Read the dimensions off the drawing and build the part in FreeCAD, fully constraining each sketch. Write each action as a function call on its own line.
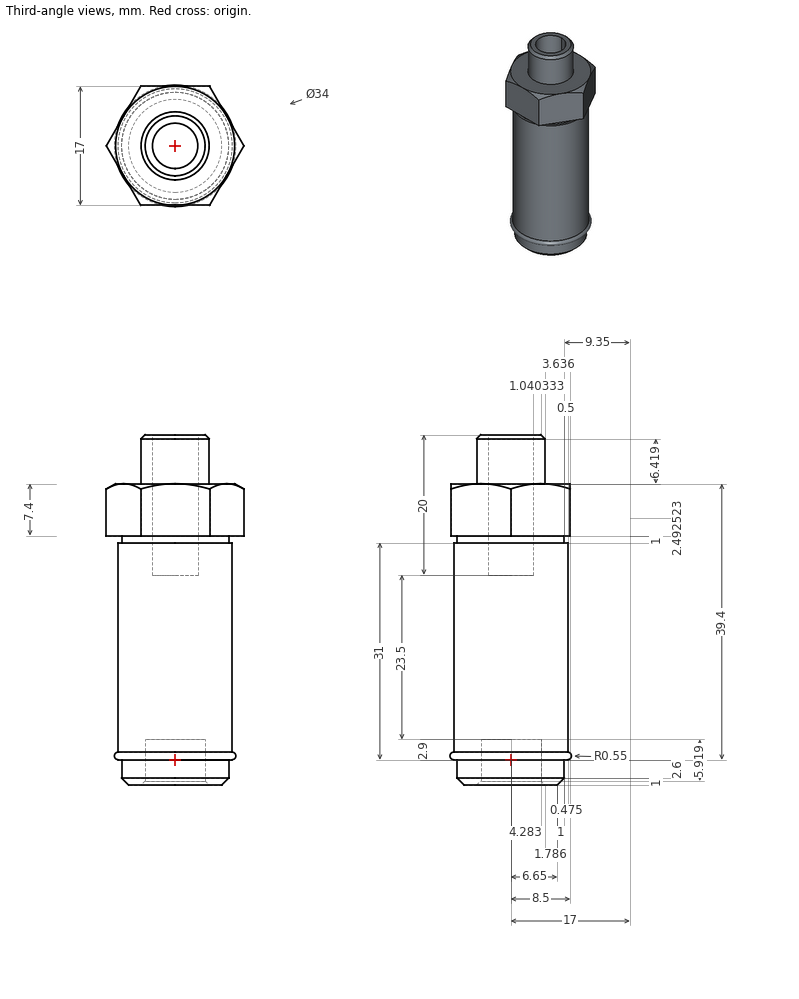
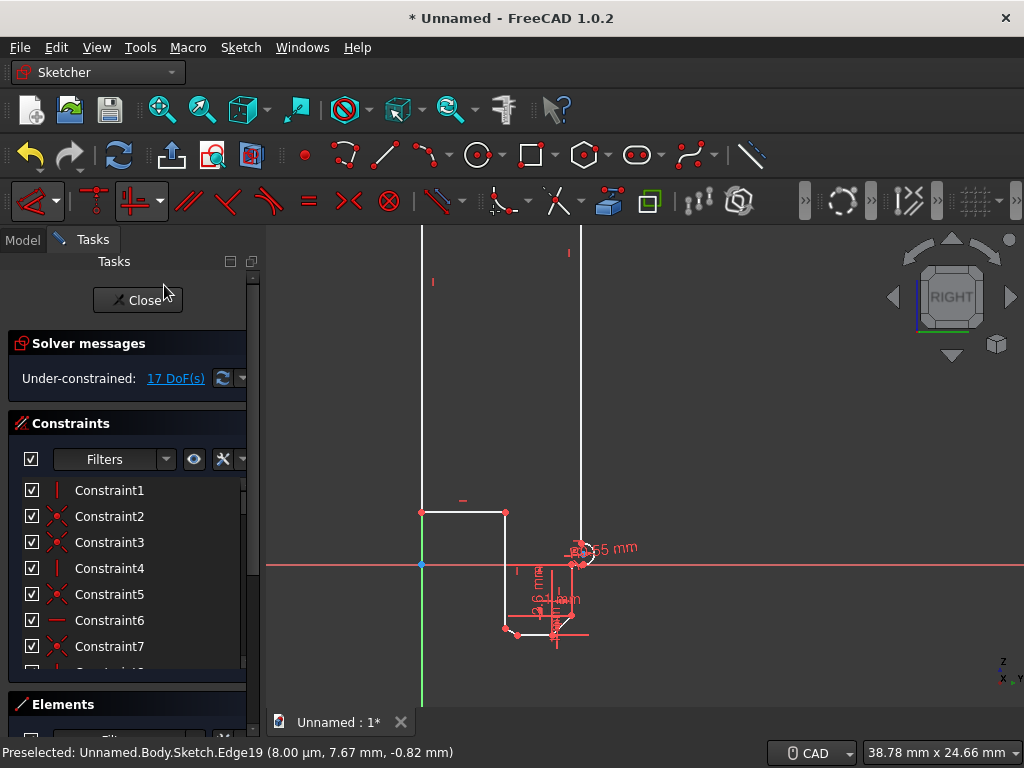
scroll(572, 604, down, 6)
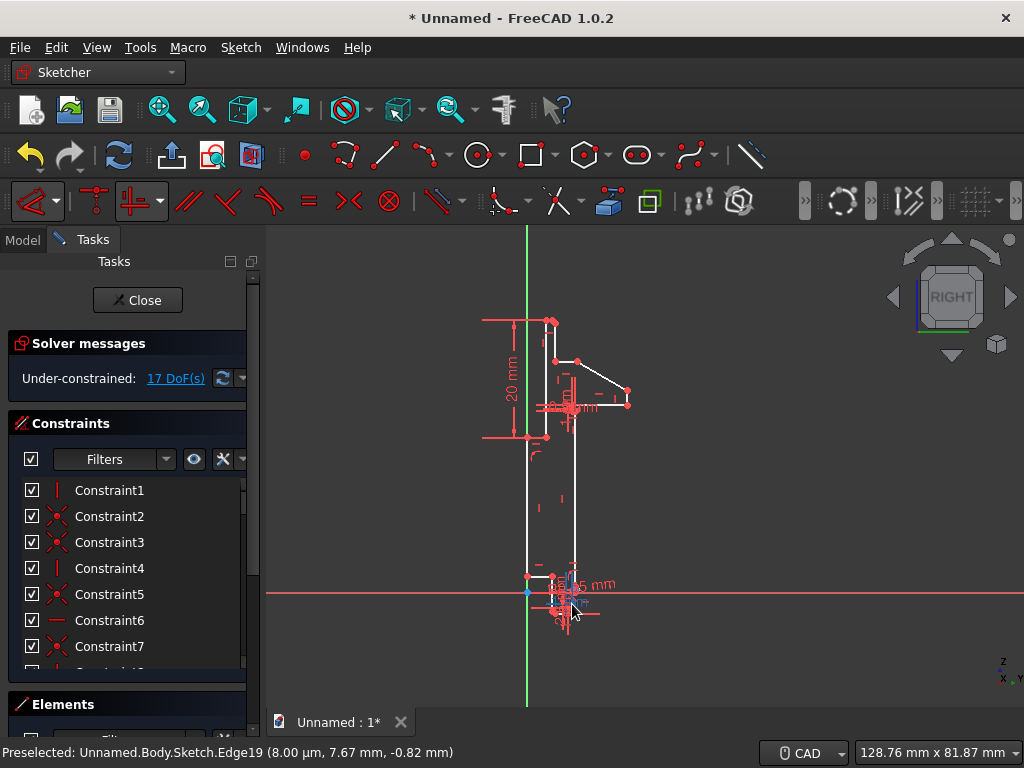
scroll(575, 411, up, 8)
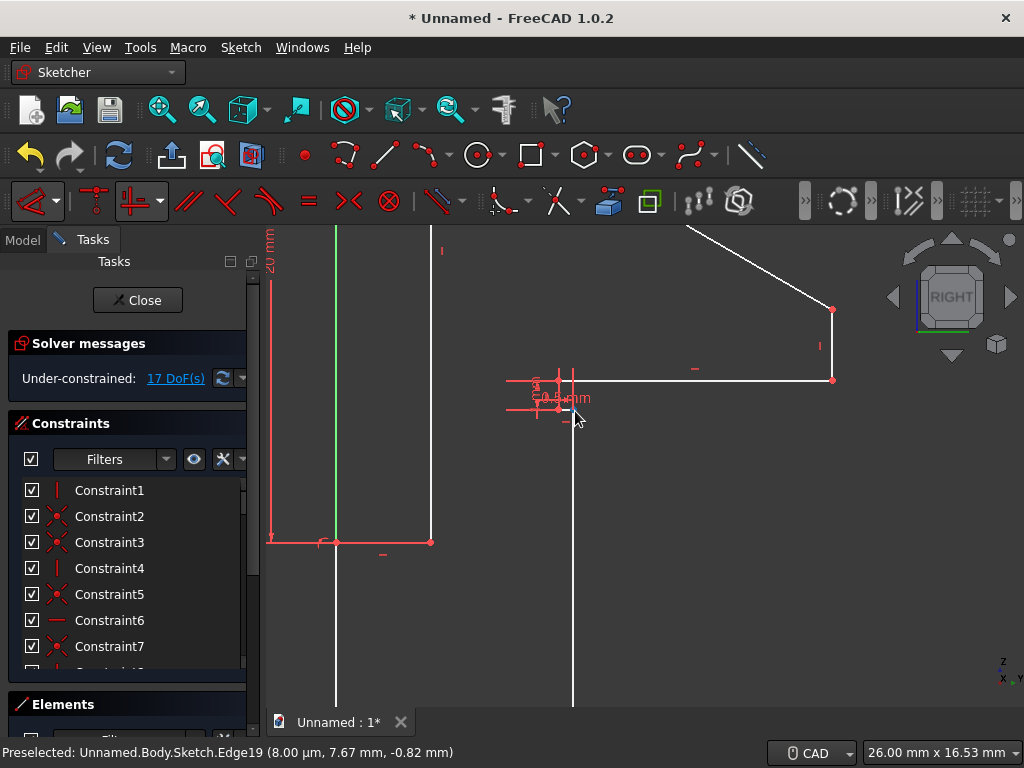
click(573, 410)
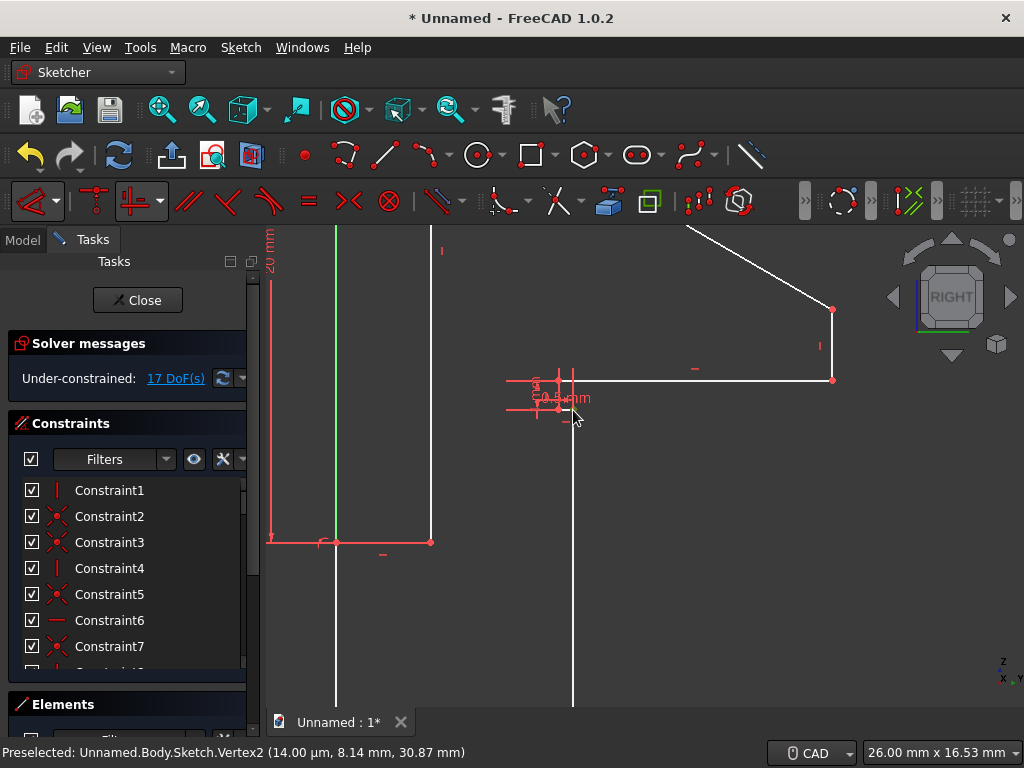
key(i)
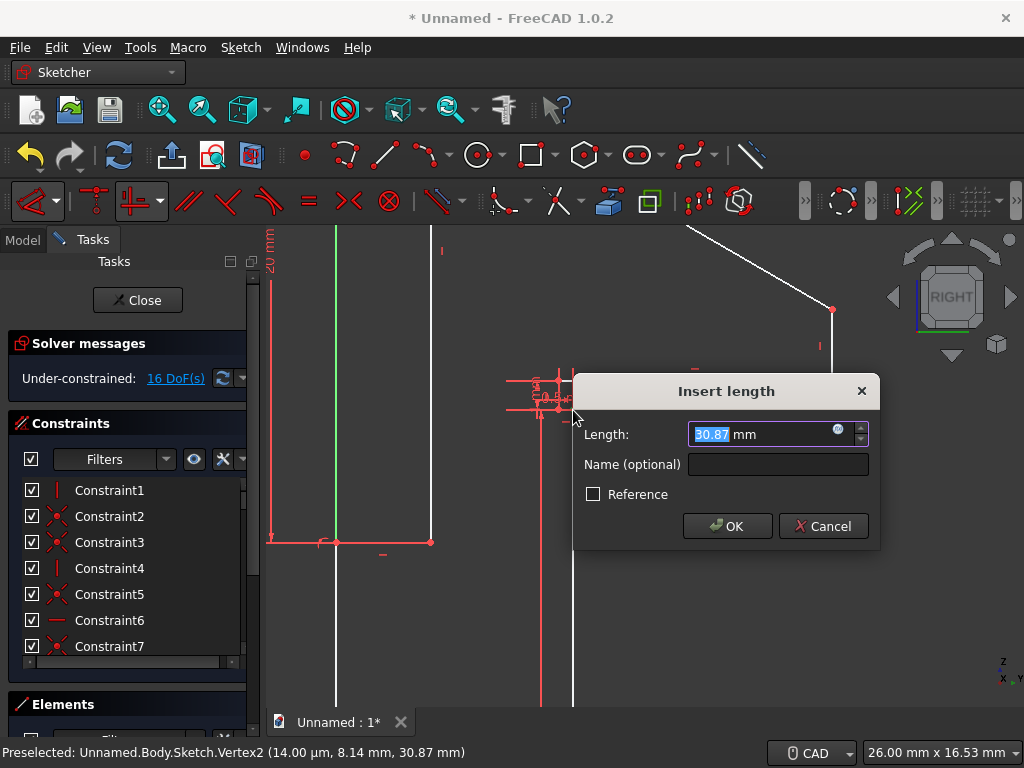
text(31)
key(Return)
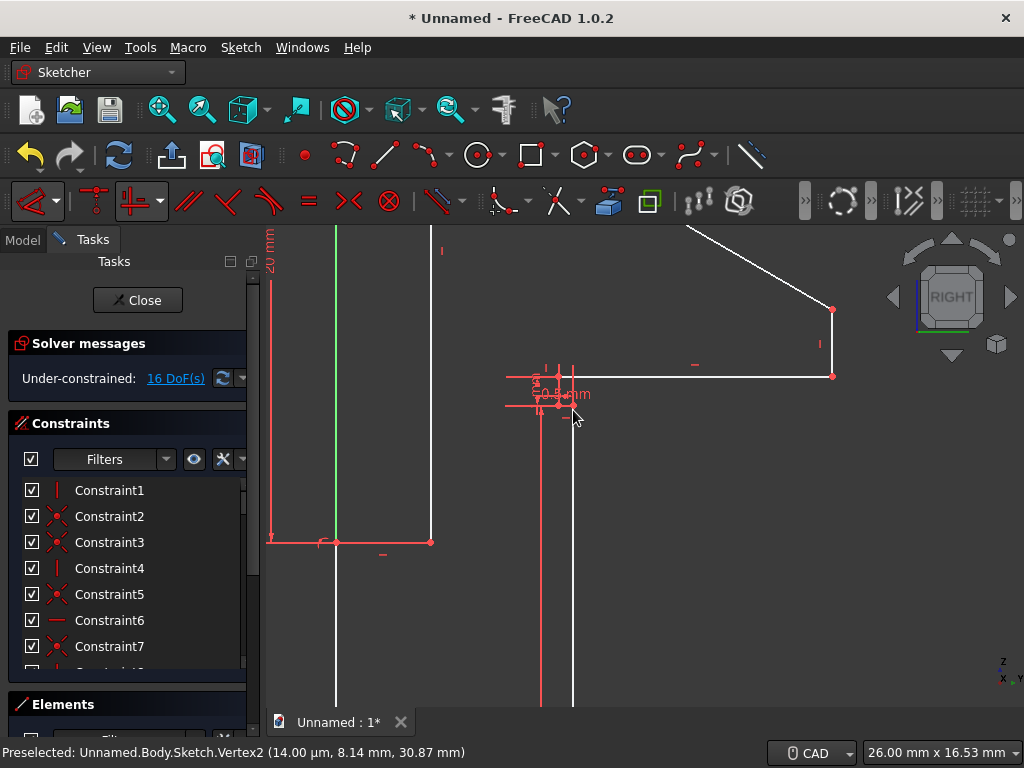
scroll(575, 410, down, 8)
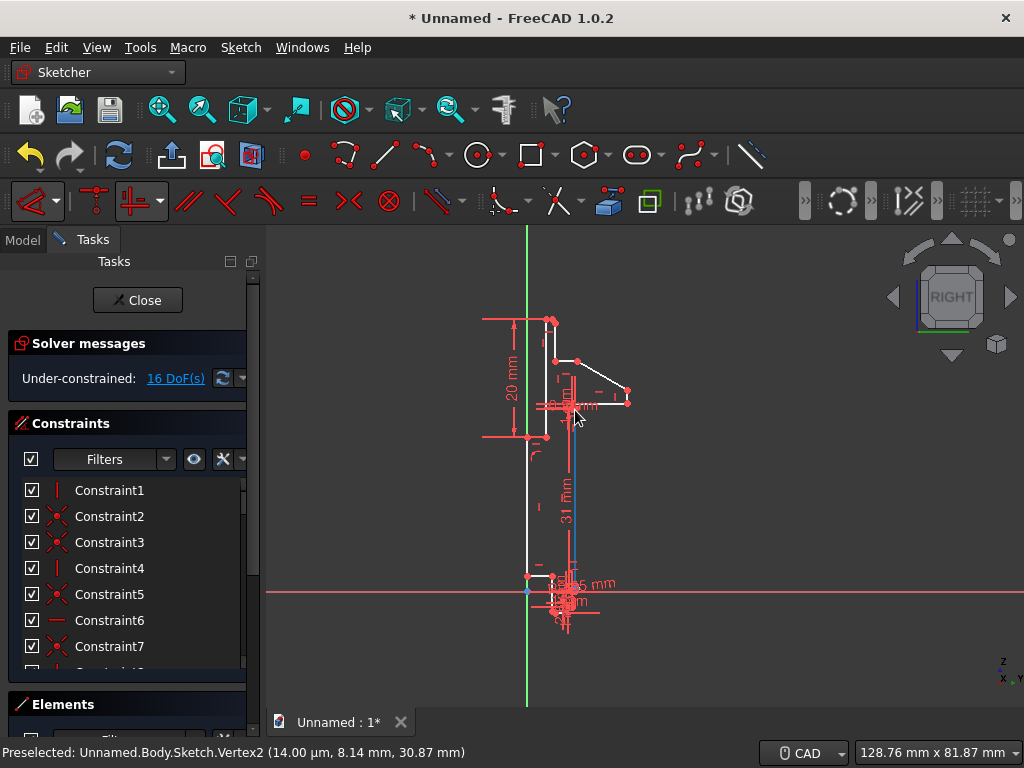
click(627, 404)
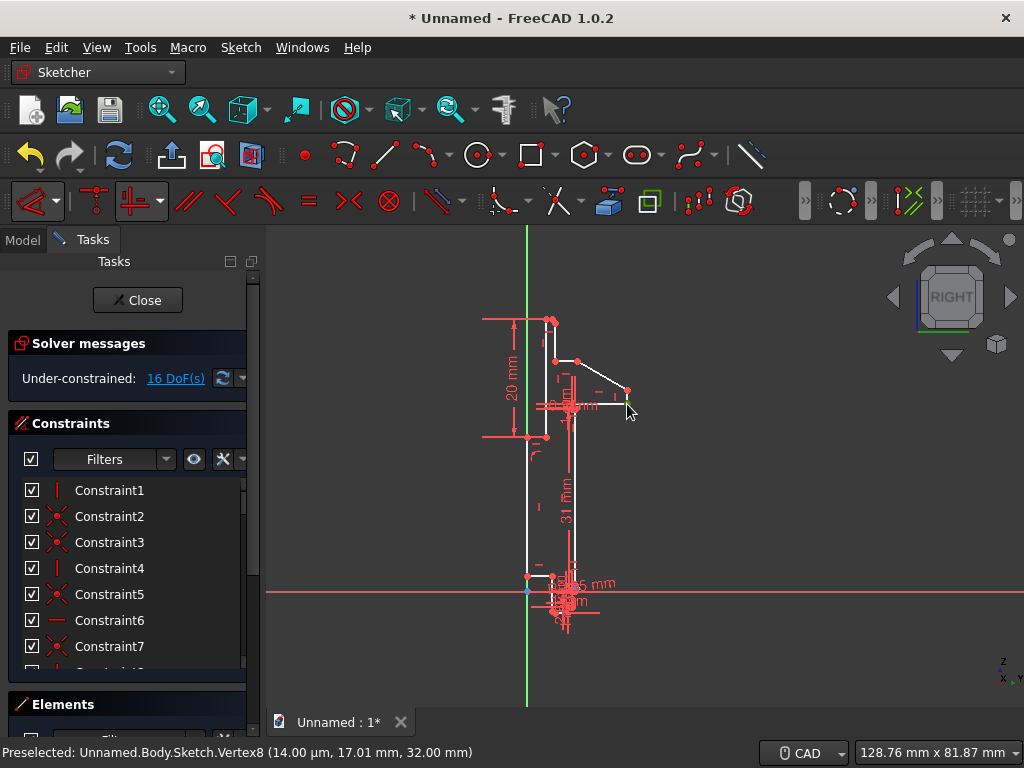
key(l)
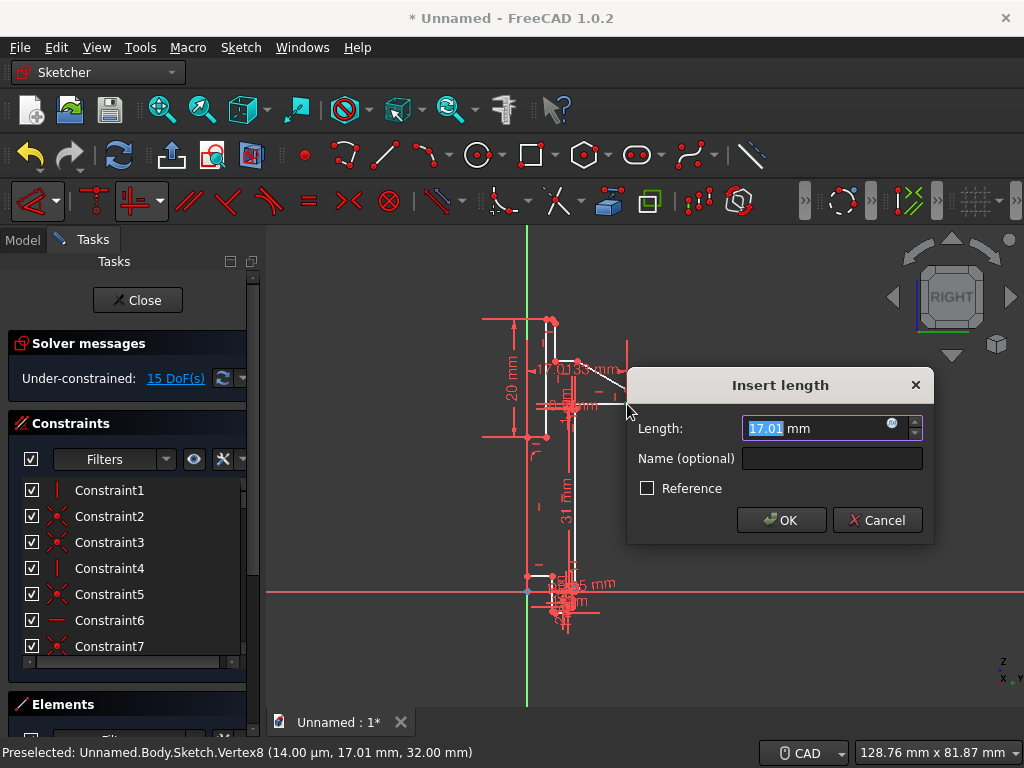
text(17)
key(Return)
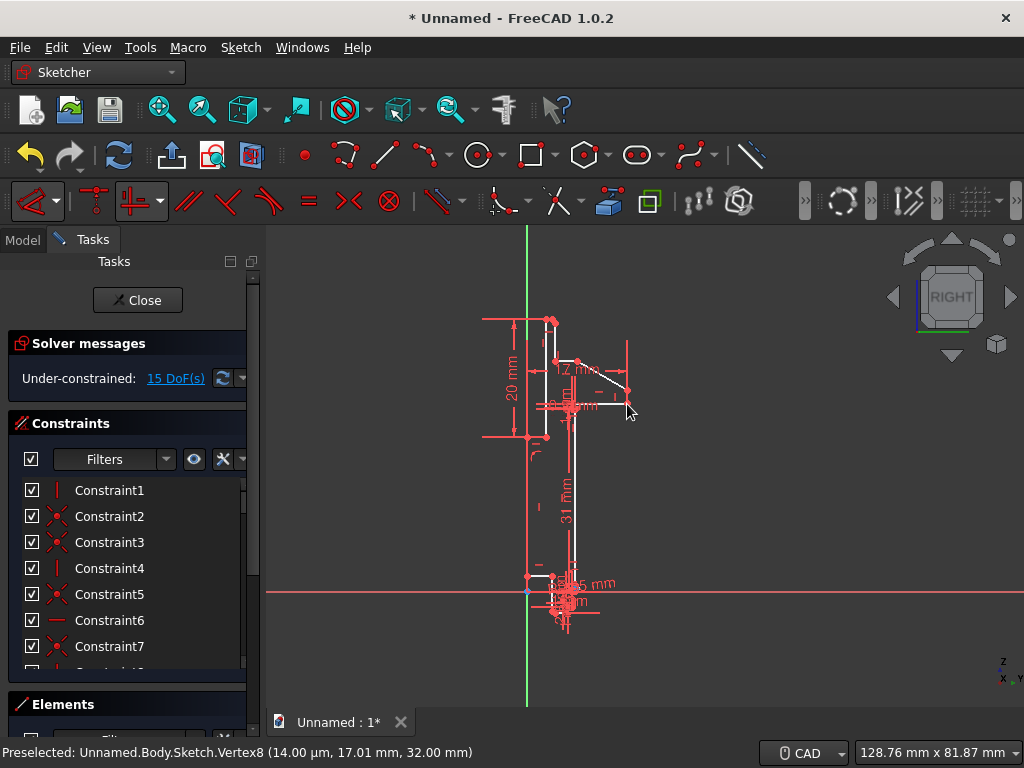
click(611, 404)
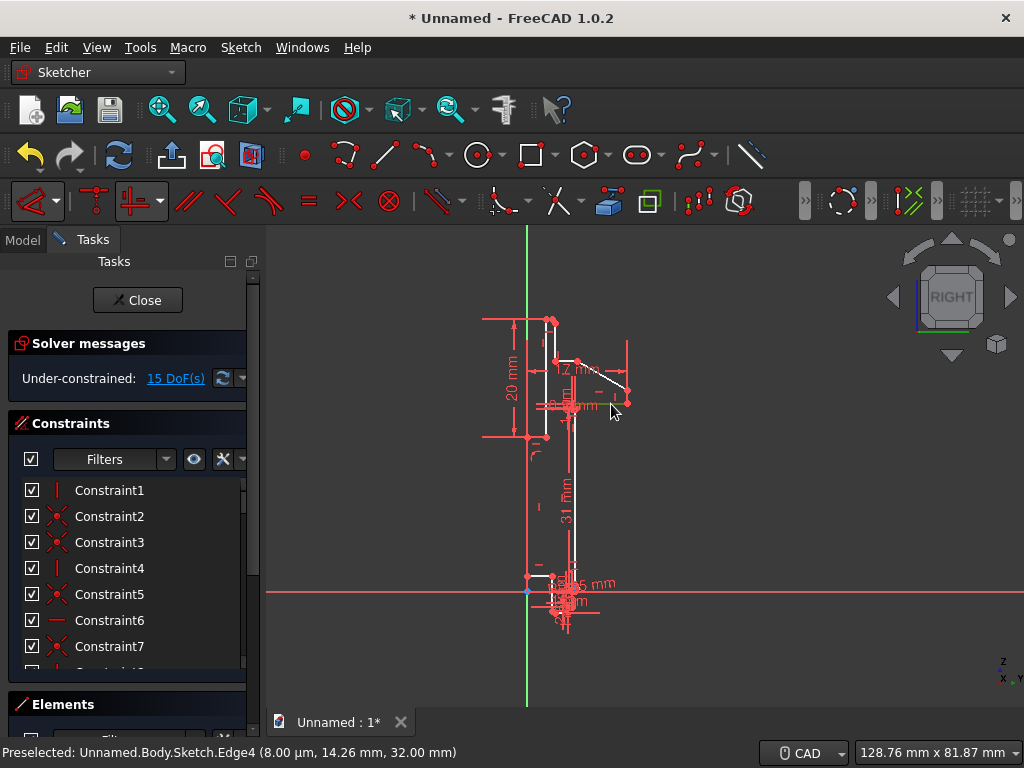
key(l)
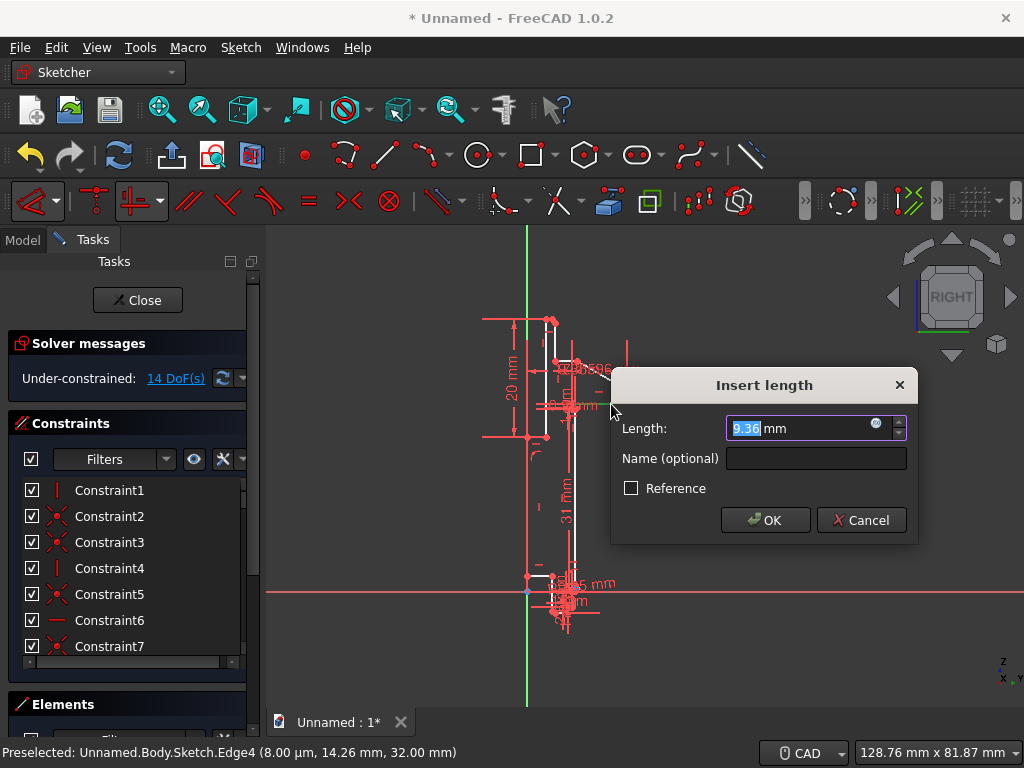
text(9.35)
key(Return)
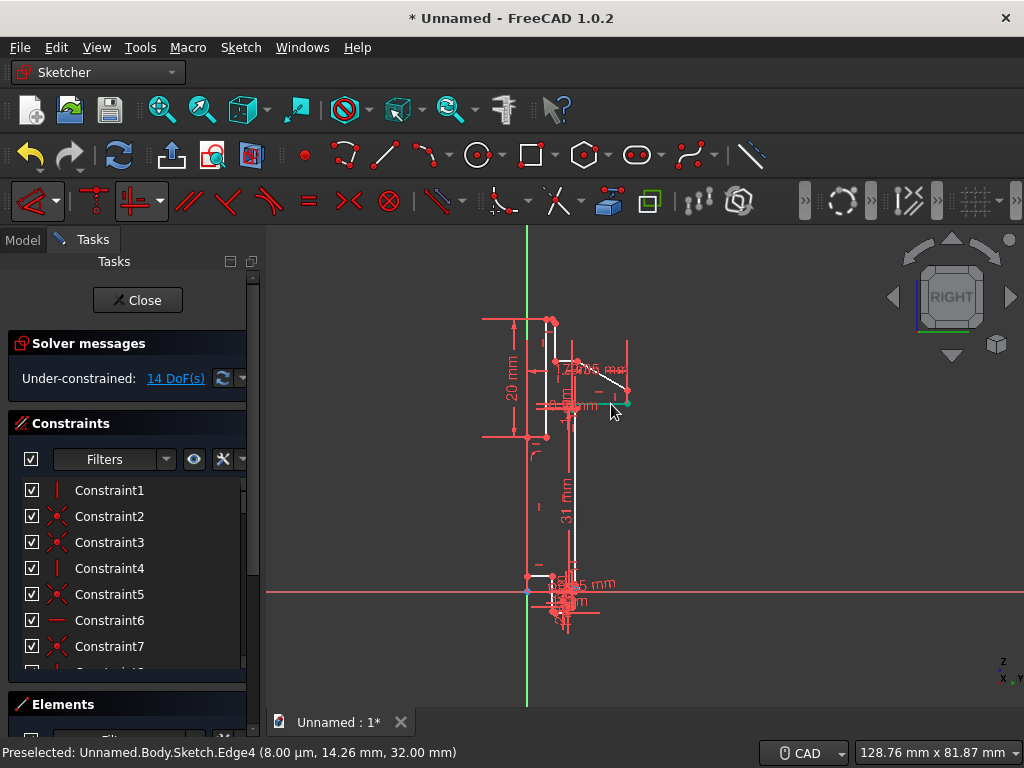
click(527, 479)